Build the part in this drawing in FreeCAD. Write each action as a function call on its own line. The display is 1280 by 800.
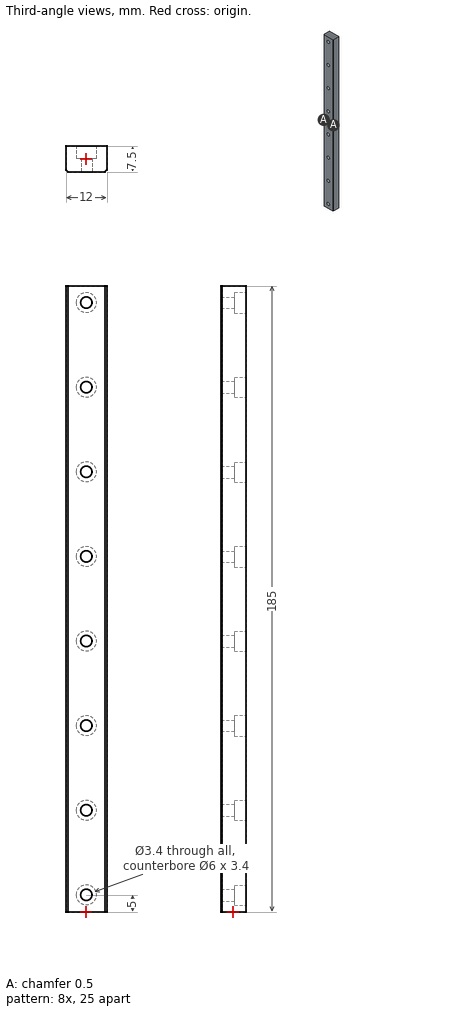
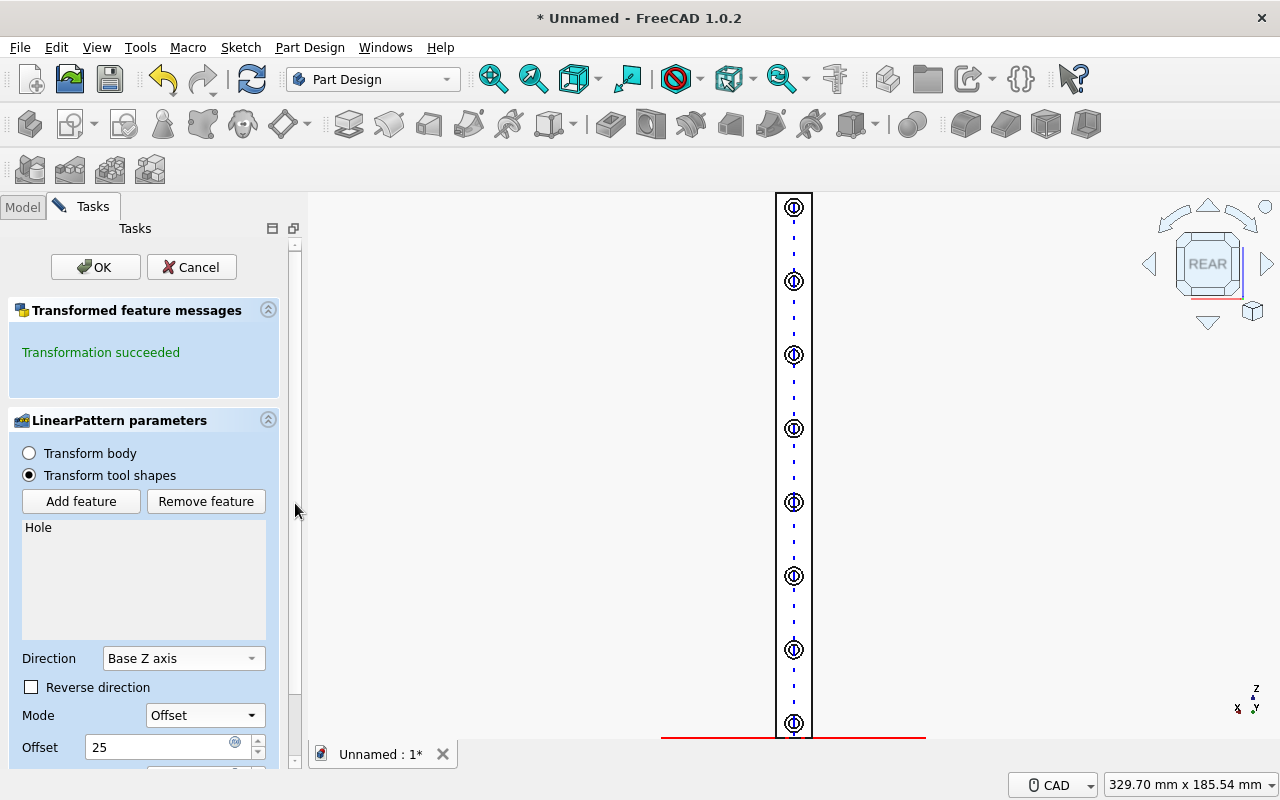
click(96, 267)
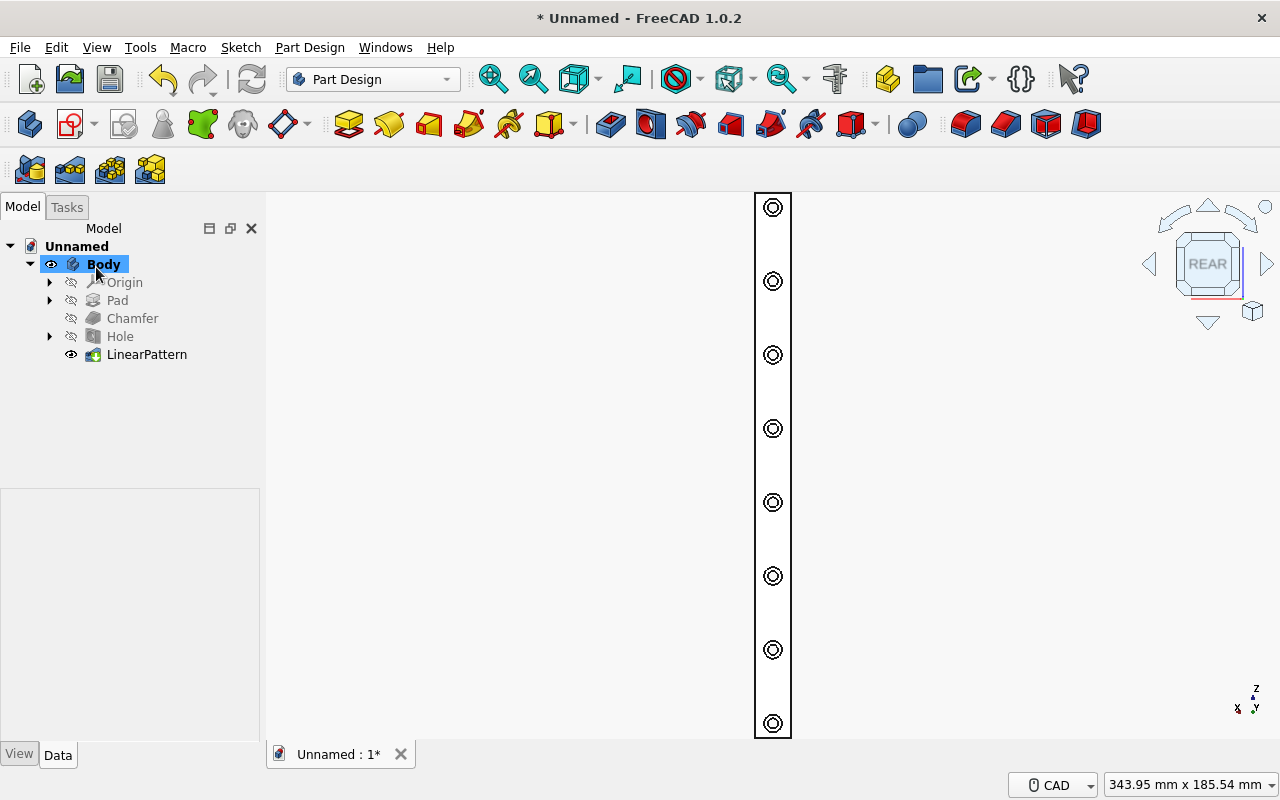
key(0)